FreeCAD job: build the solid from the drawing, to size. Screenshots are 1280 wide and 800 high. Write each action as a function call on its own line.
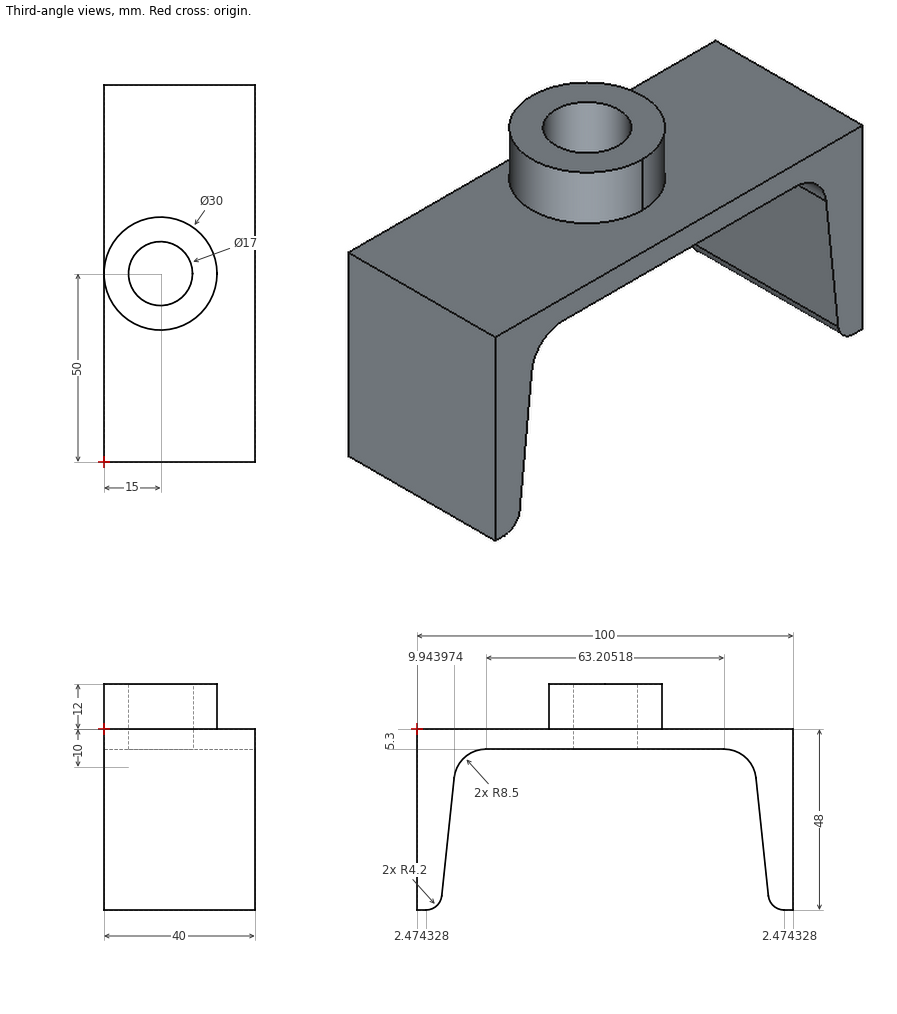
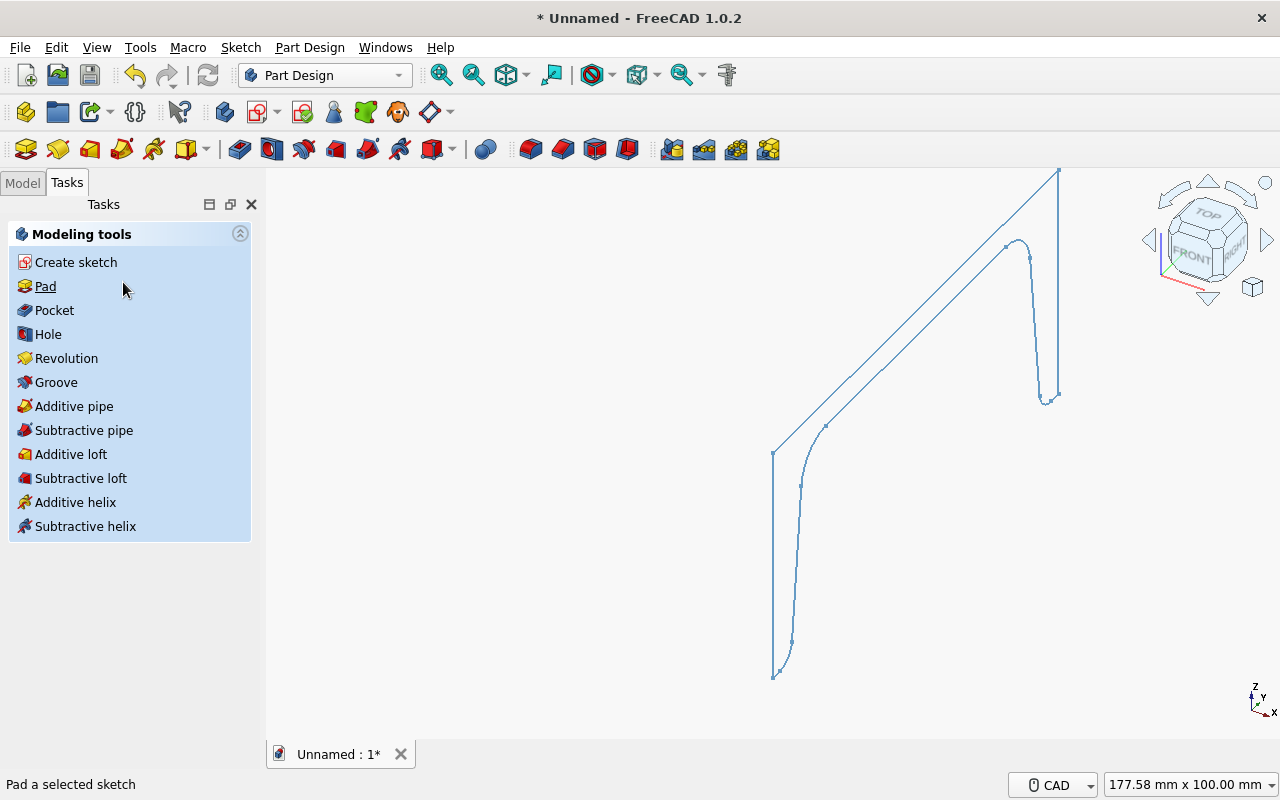
click(26, 150)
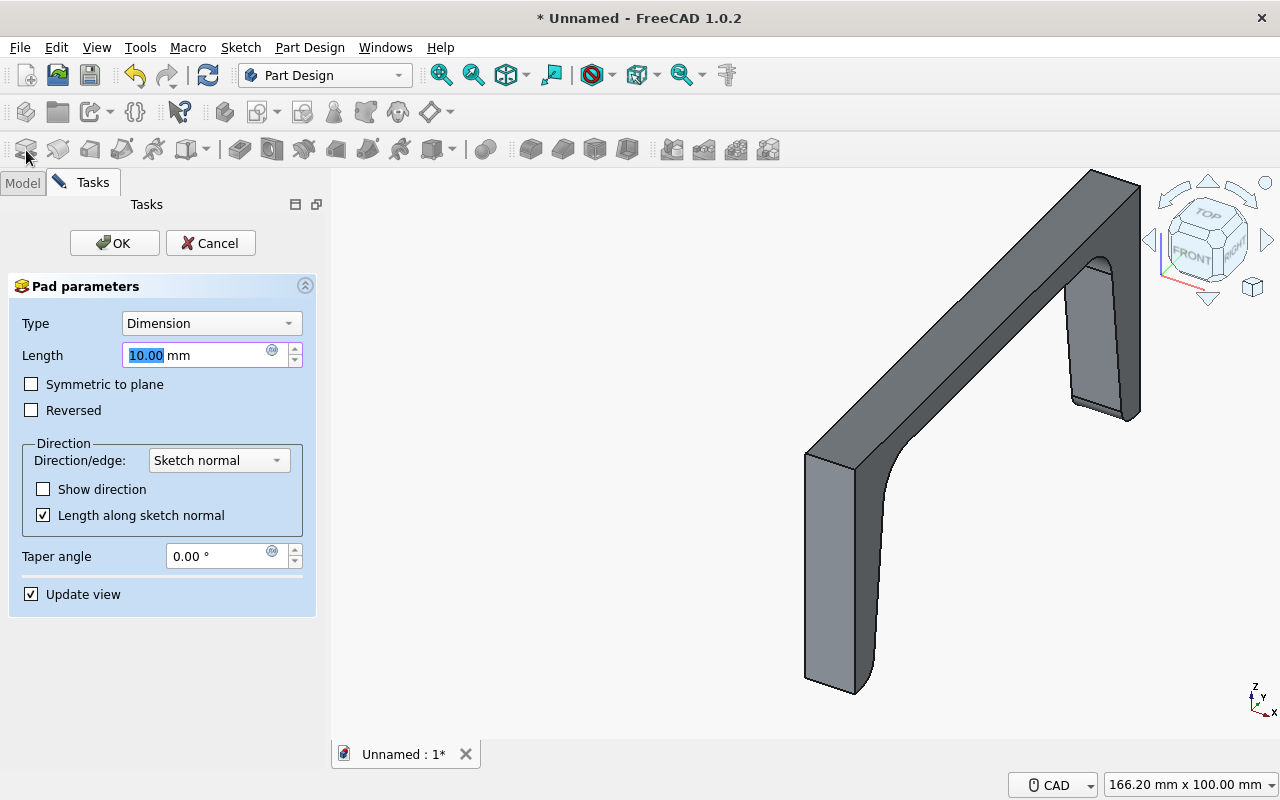
text(40)
key(Tab)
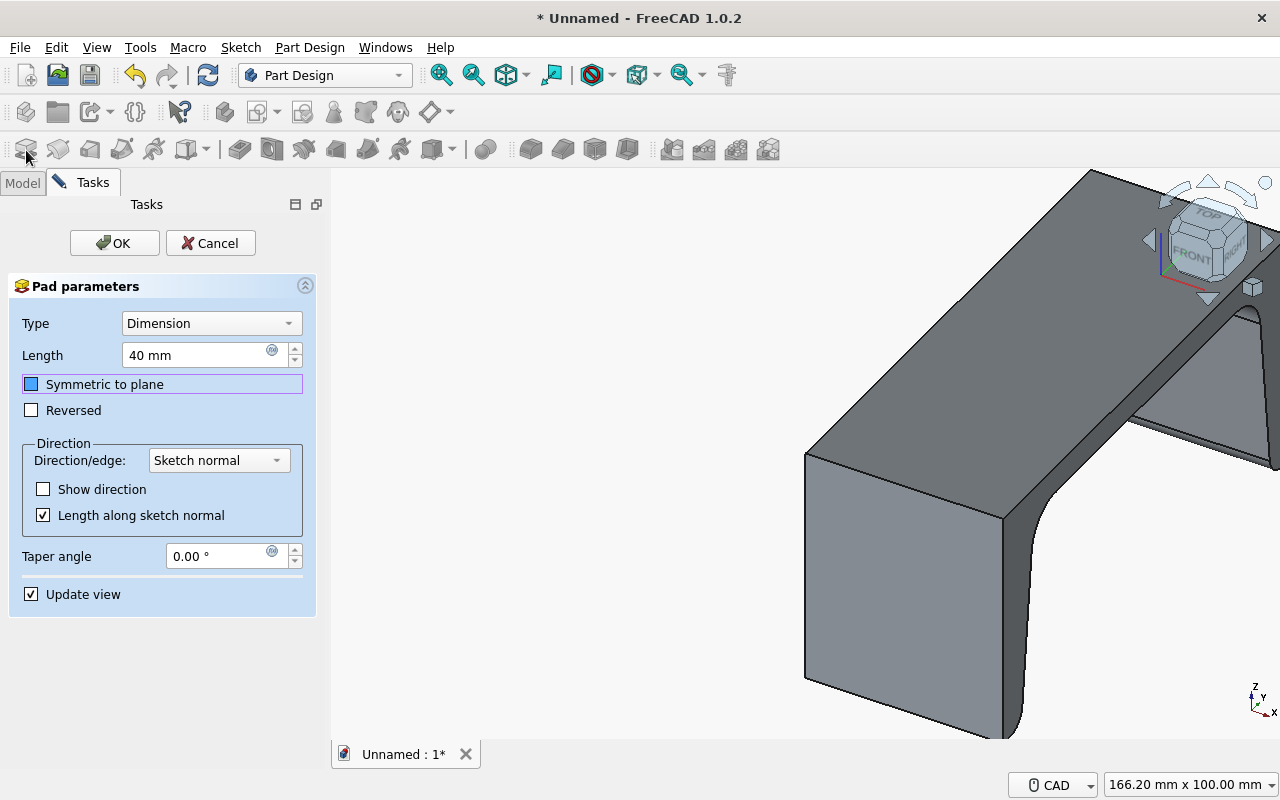
click(115, 243)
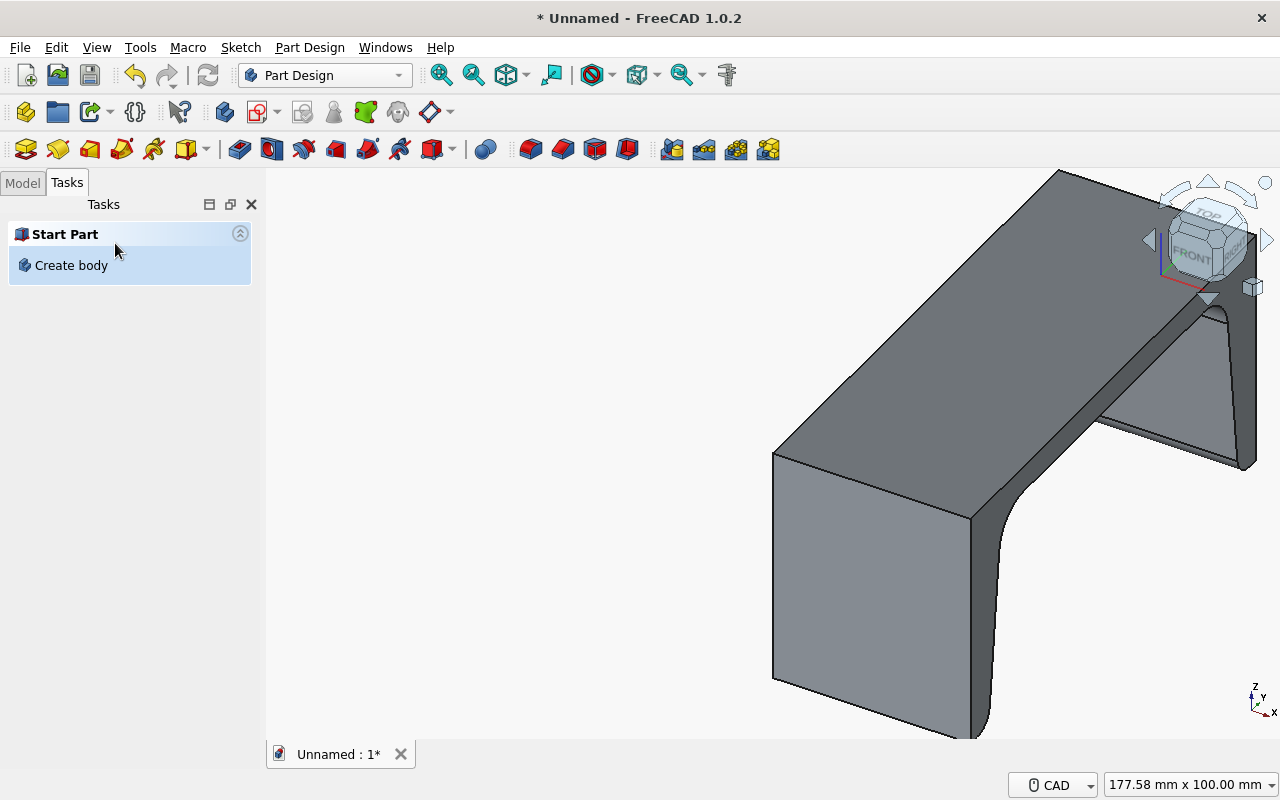
click(442, 76)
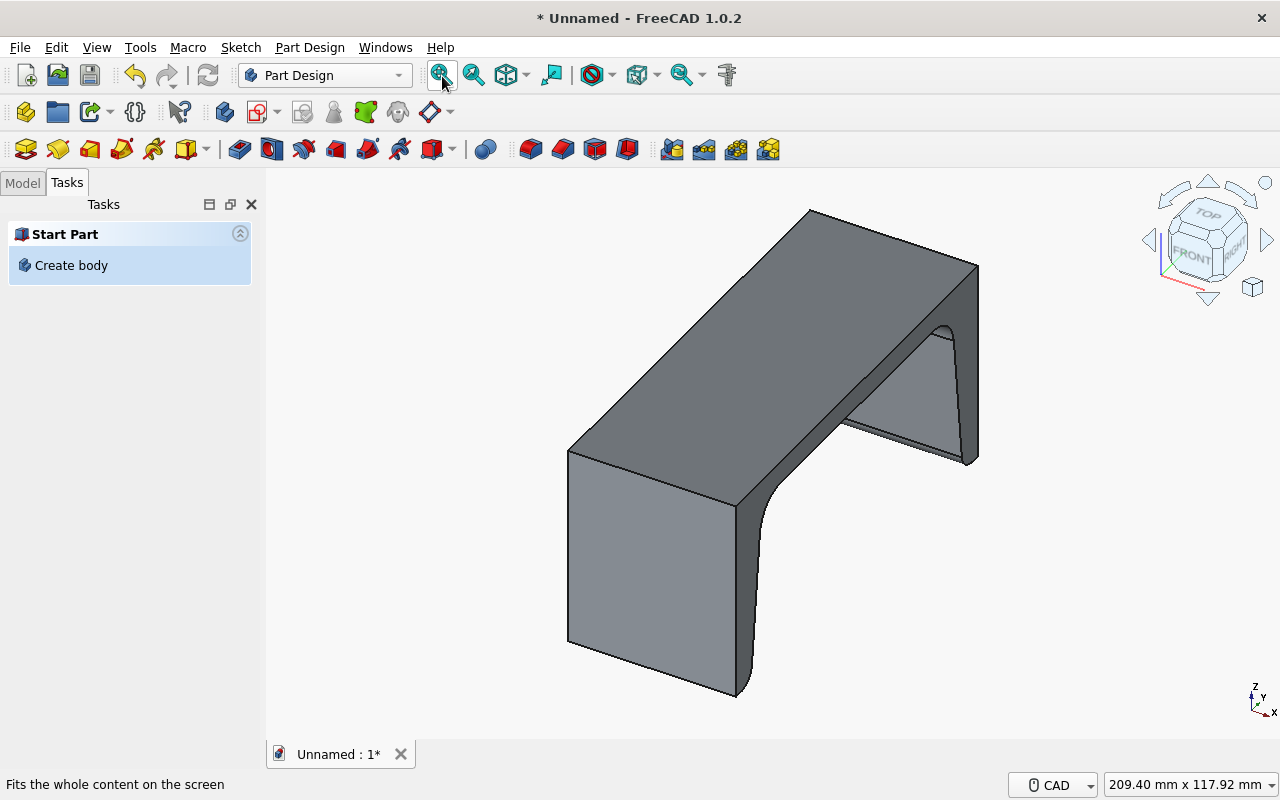
click(842, 289)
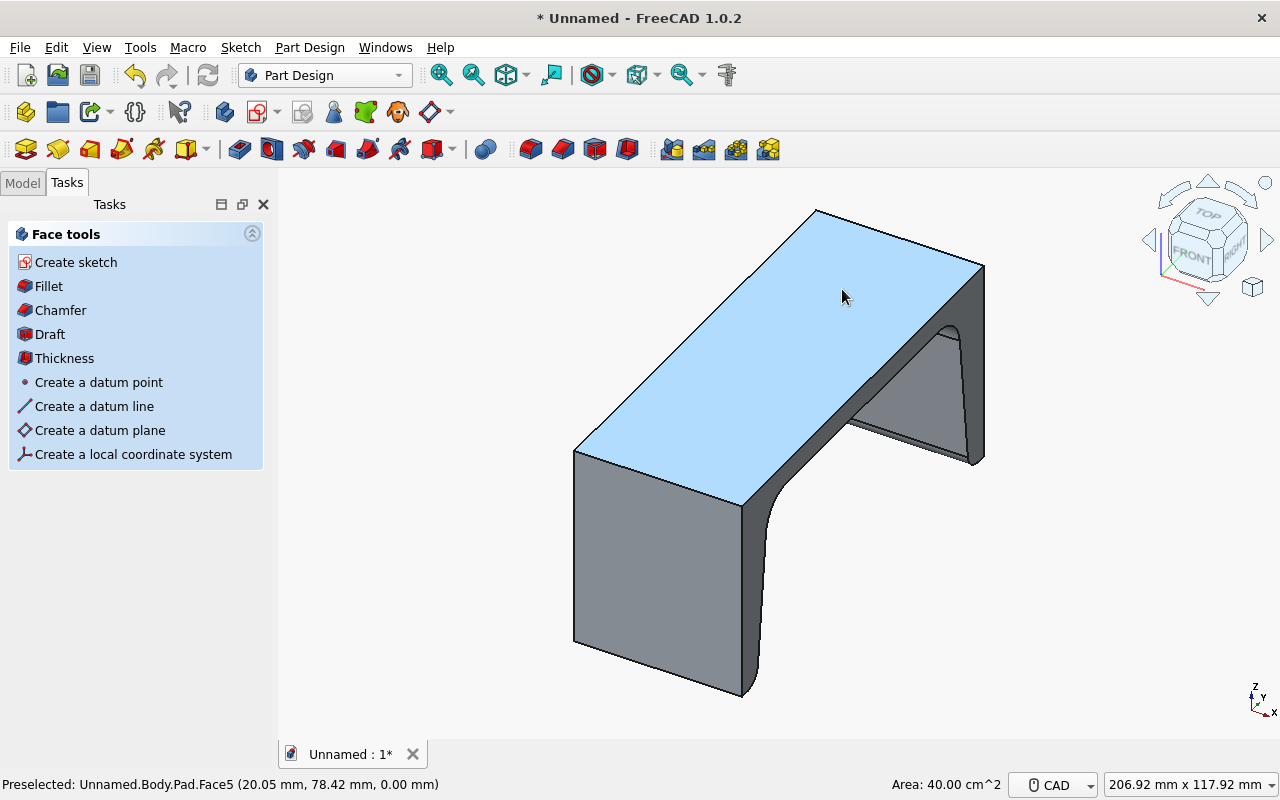
click(258, 112)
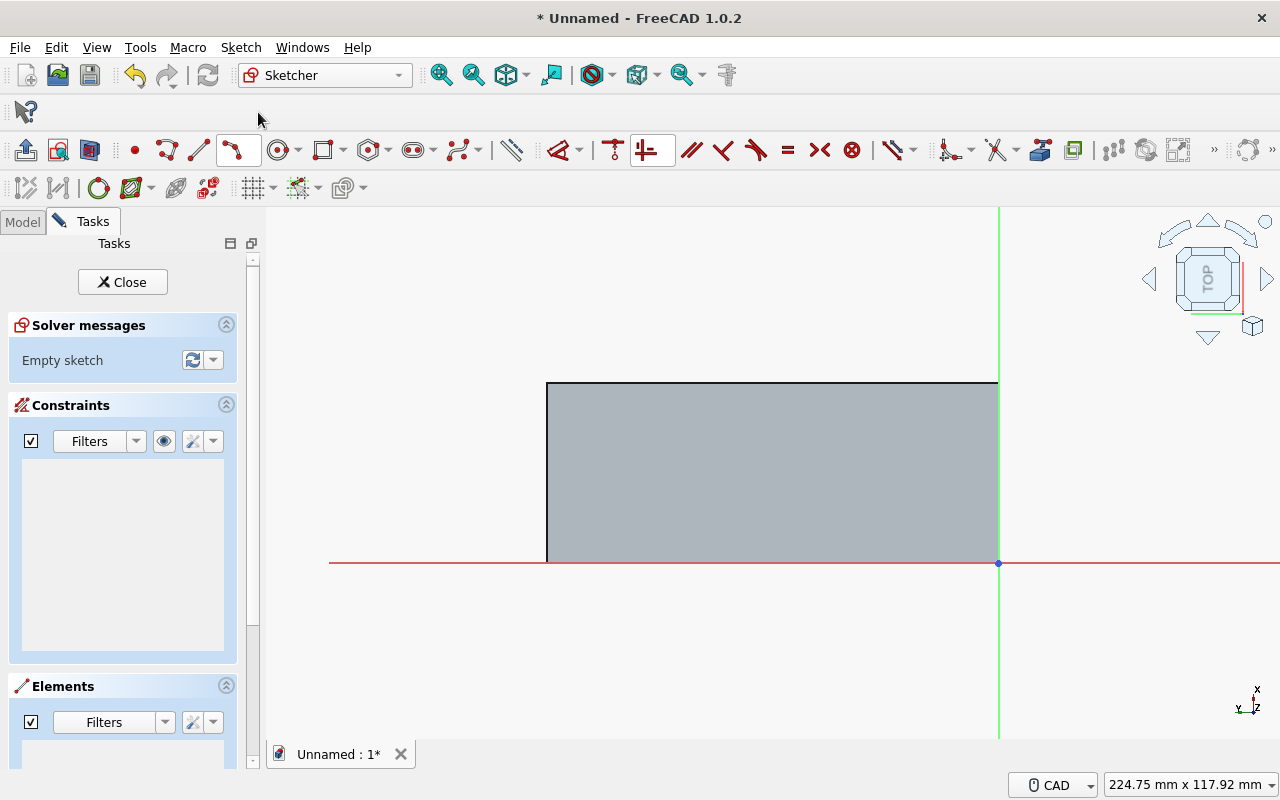
scroll(795, 503, up, 7)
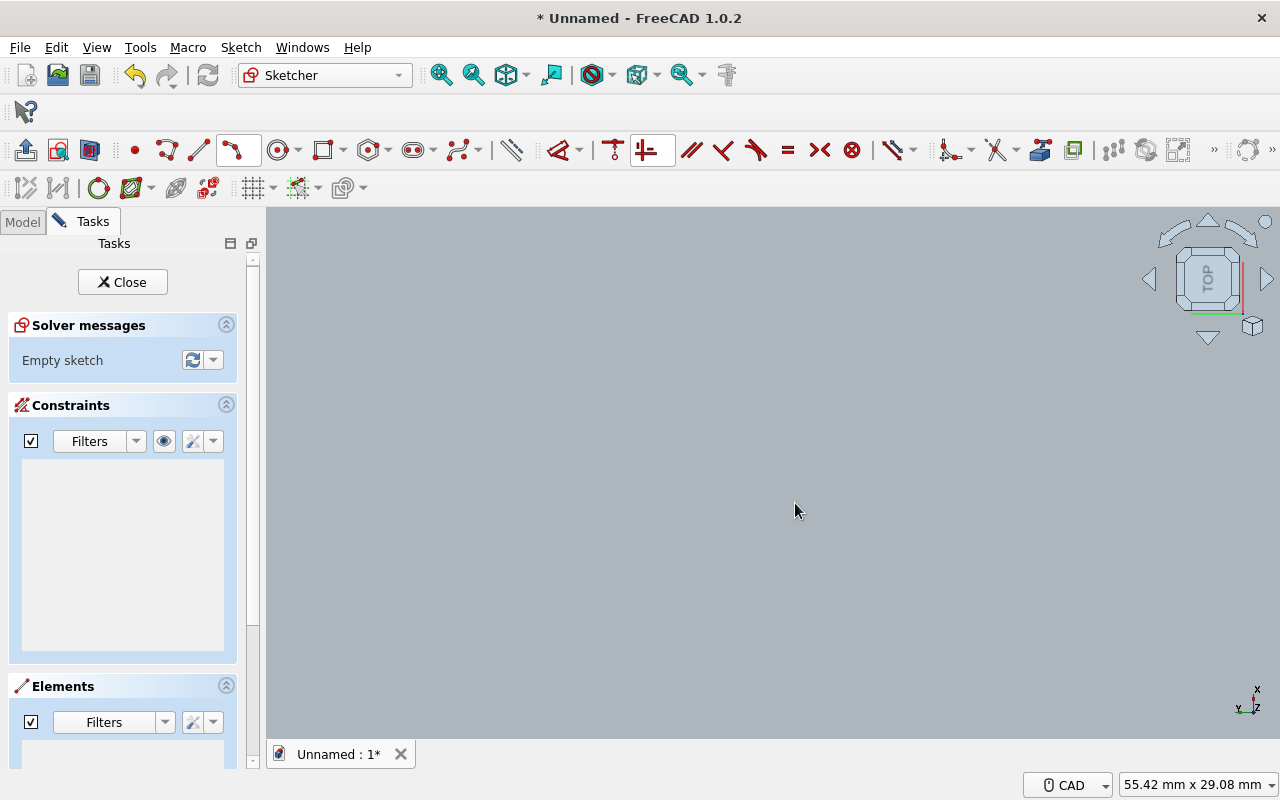
click(278, 150)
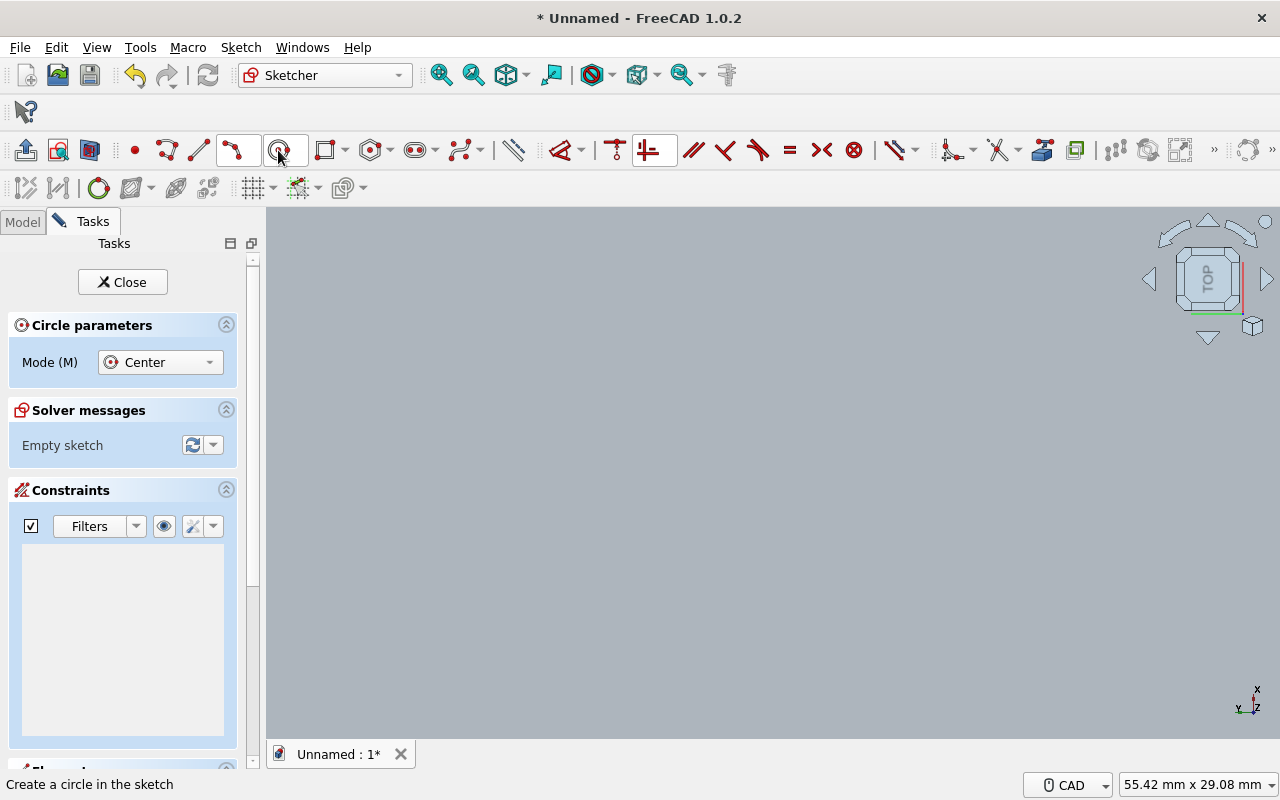
click(704, 471)
move(814, 361)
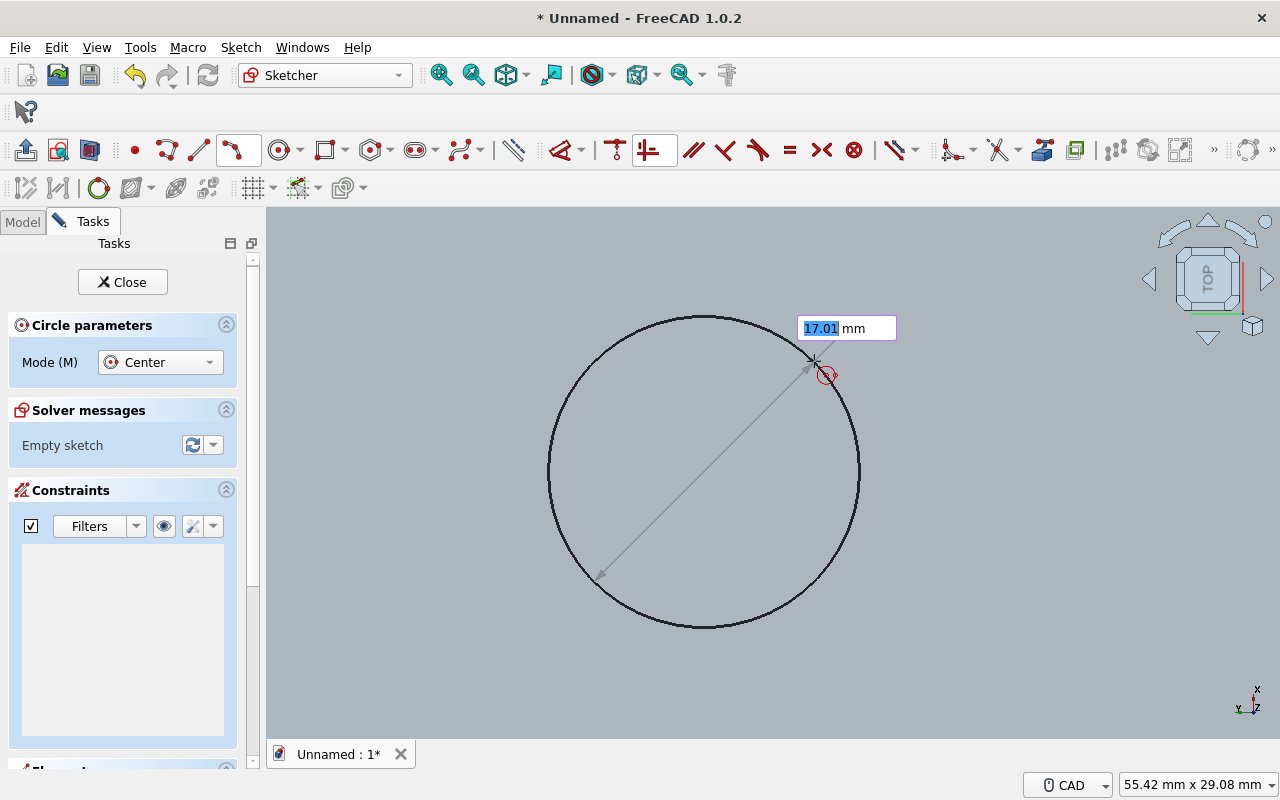
text(17)
key(Return)
key(Escape)